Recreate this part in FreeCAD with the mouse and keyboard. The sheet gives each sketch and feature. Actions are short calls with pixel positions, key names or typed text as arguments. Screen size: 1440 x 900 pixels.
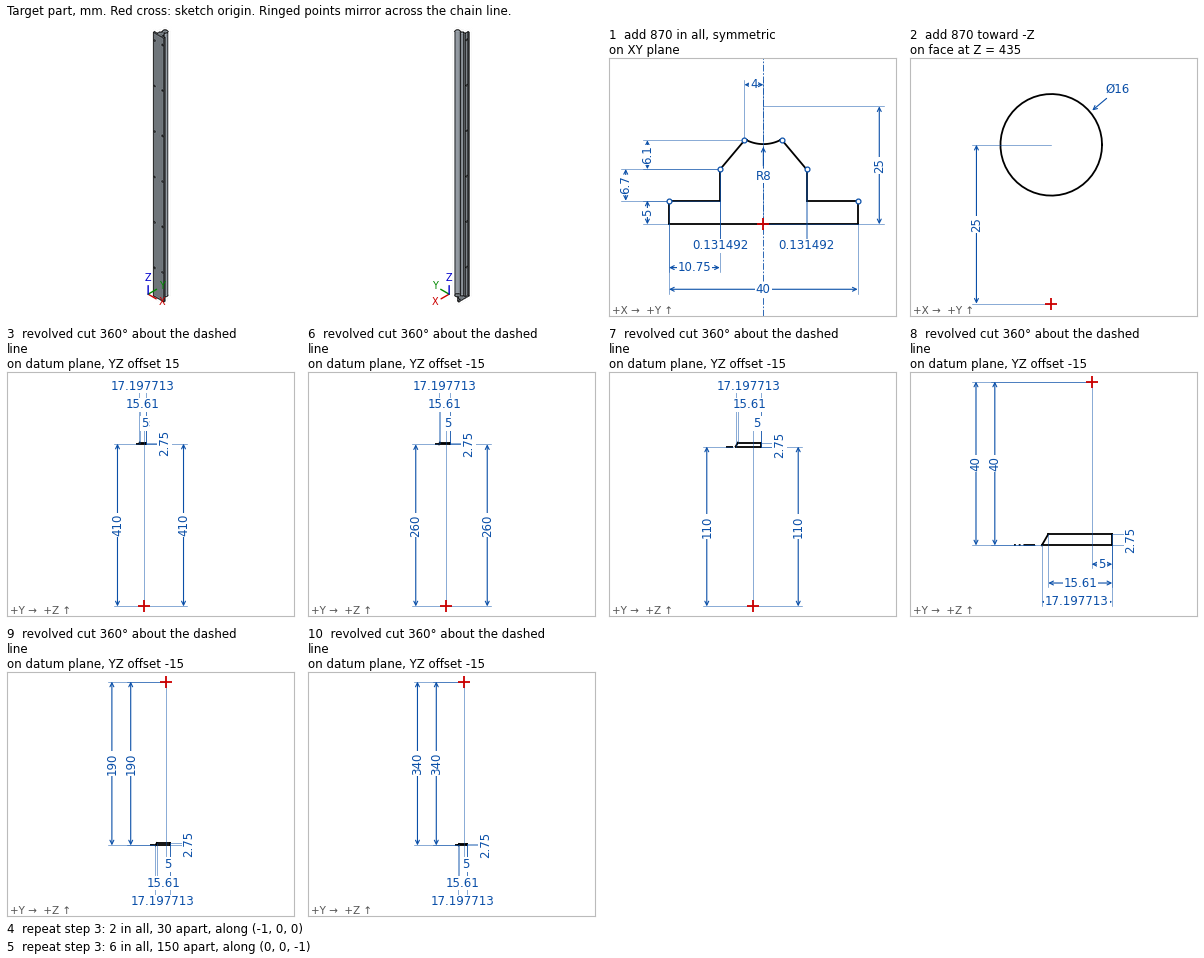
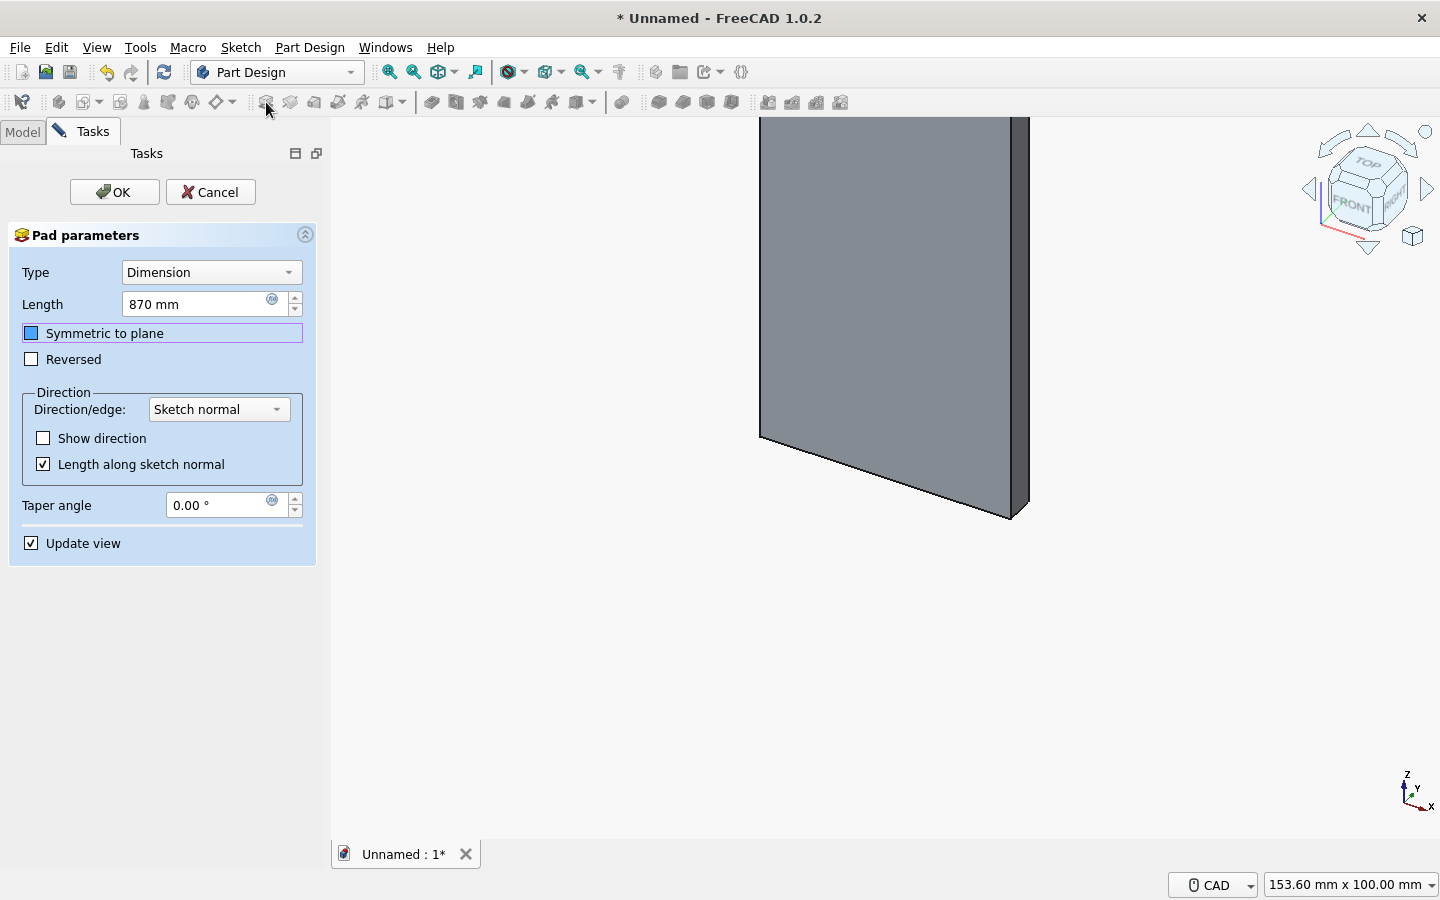
click(30, 333)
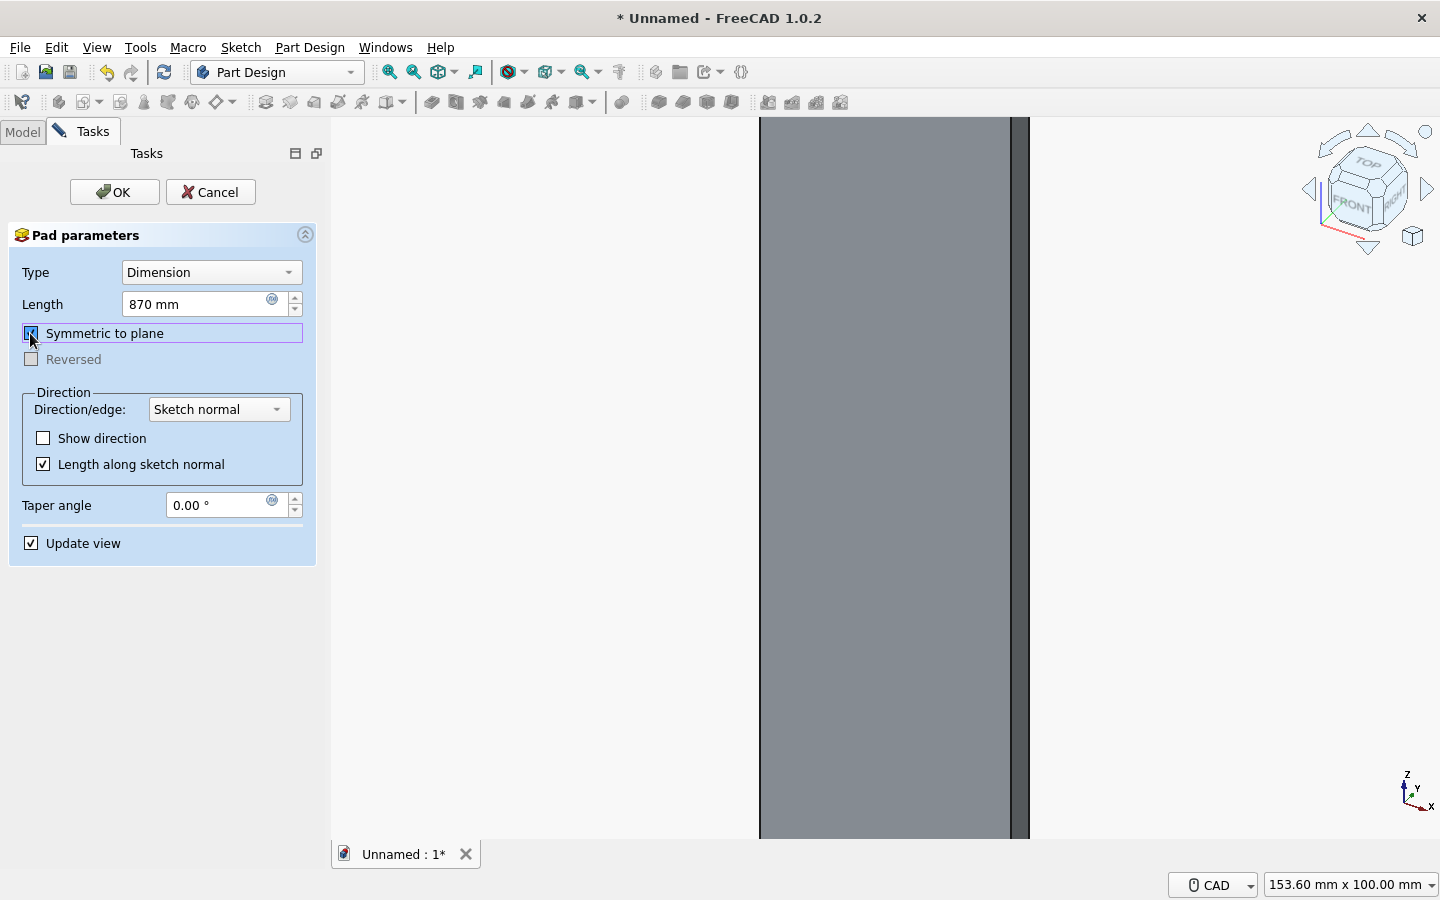
click(115, 192)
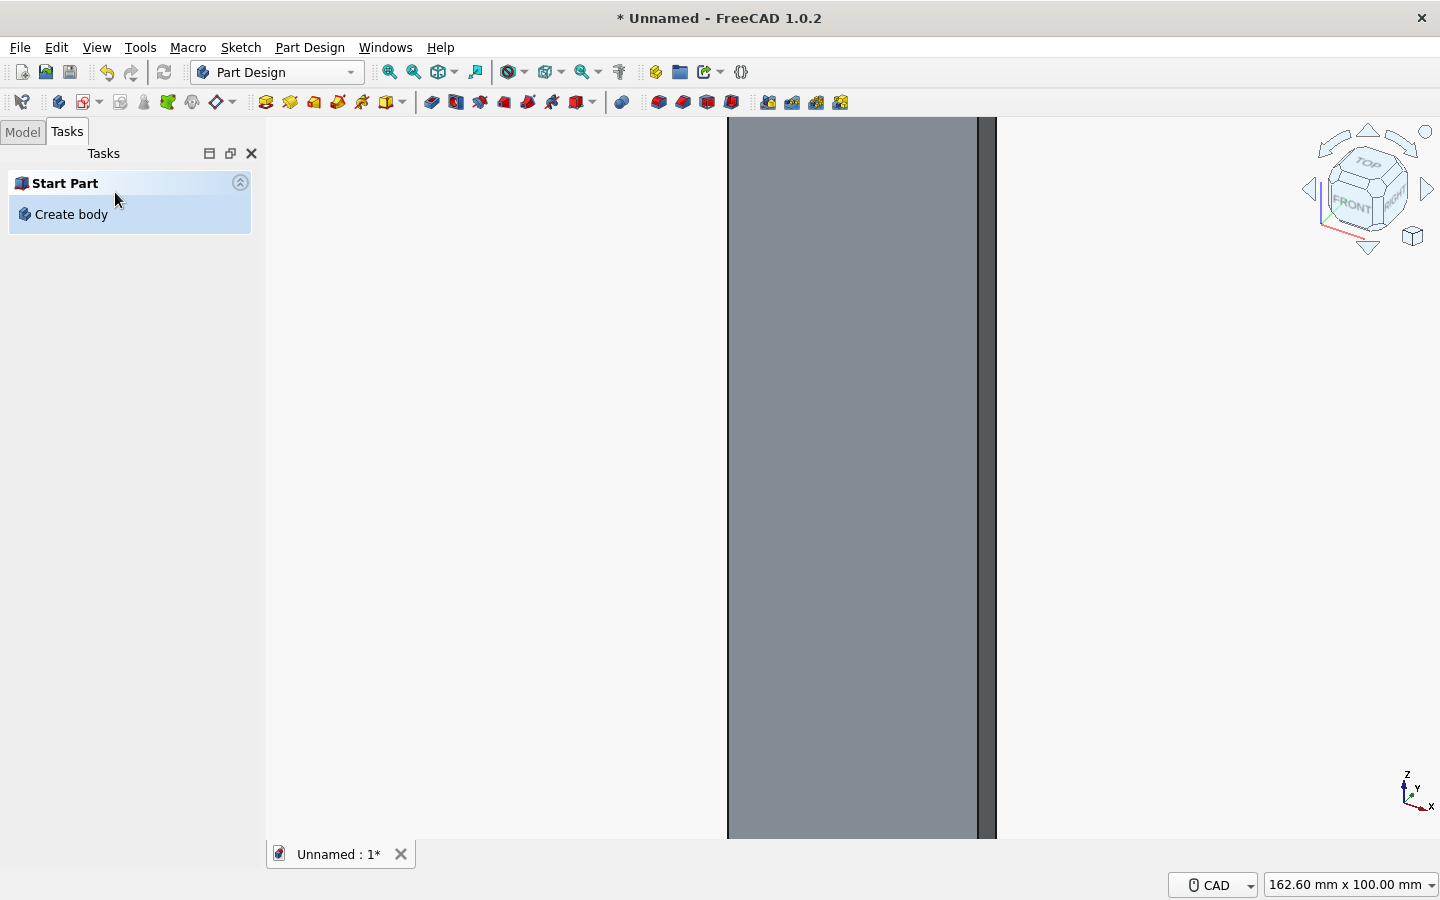
click(390, 72)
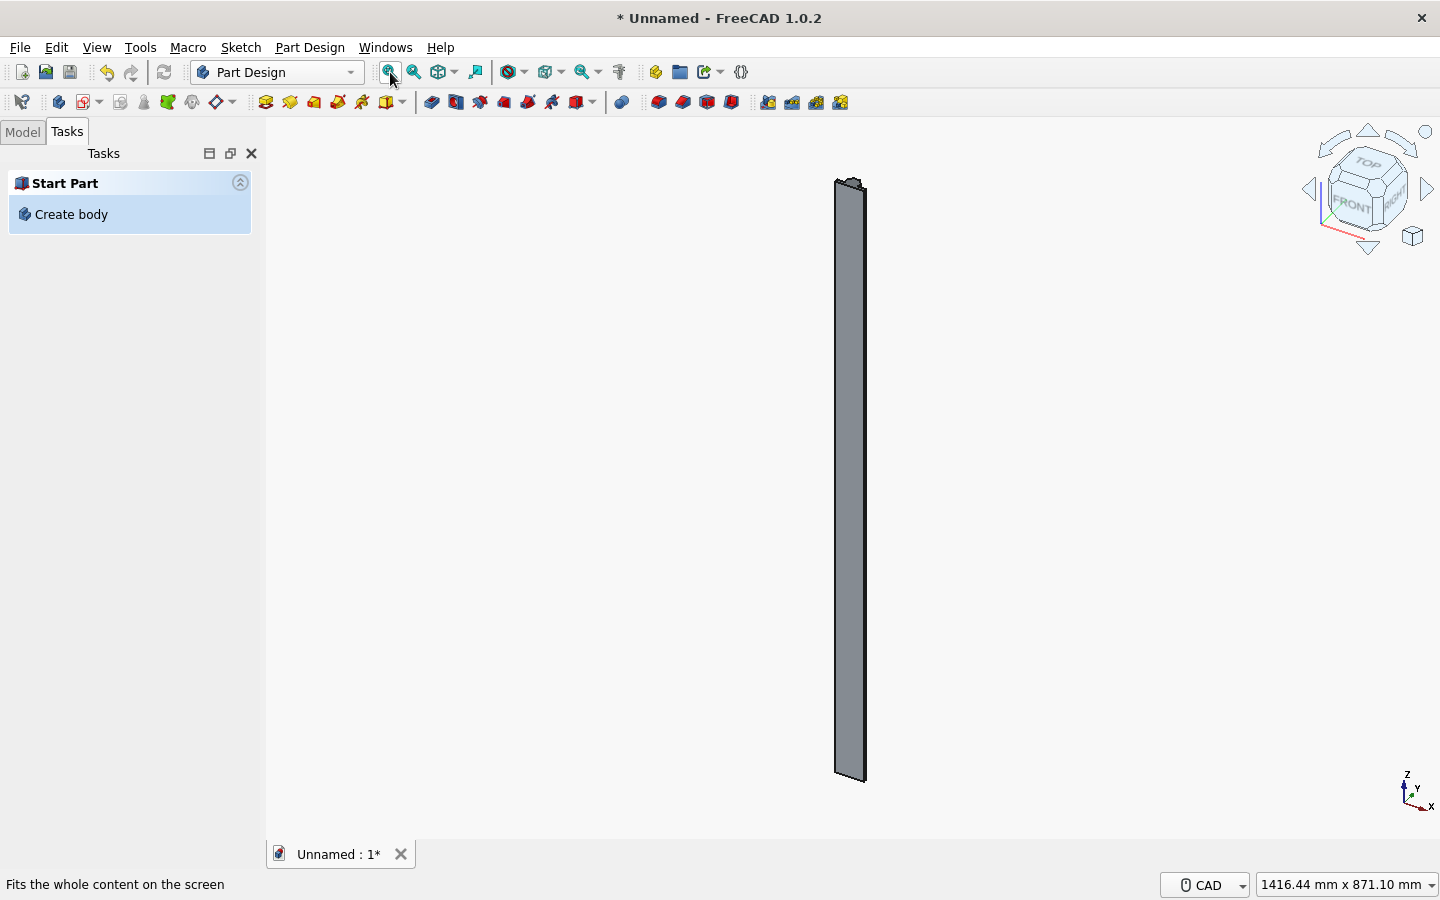
scroll(853, 182, up, 3)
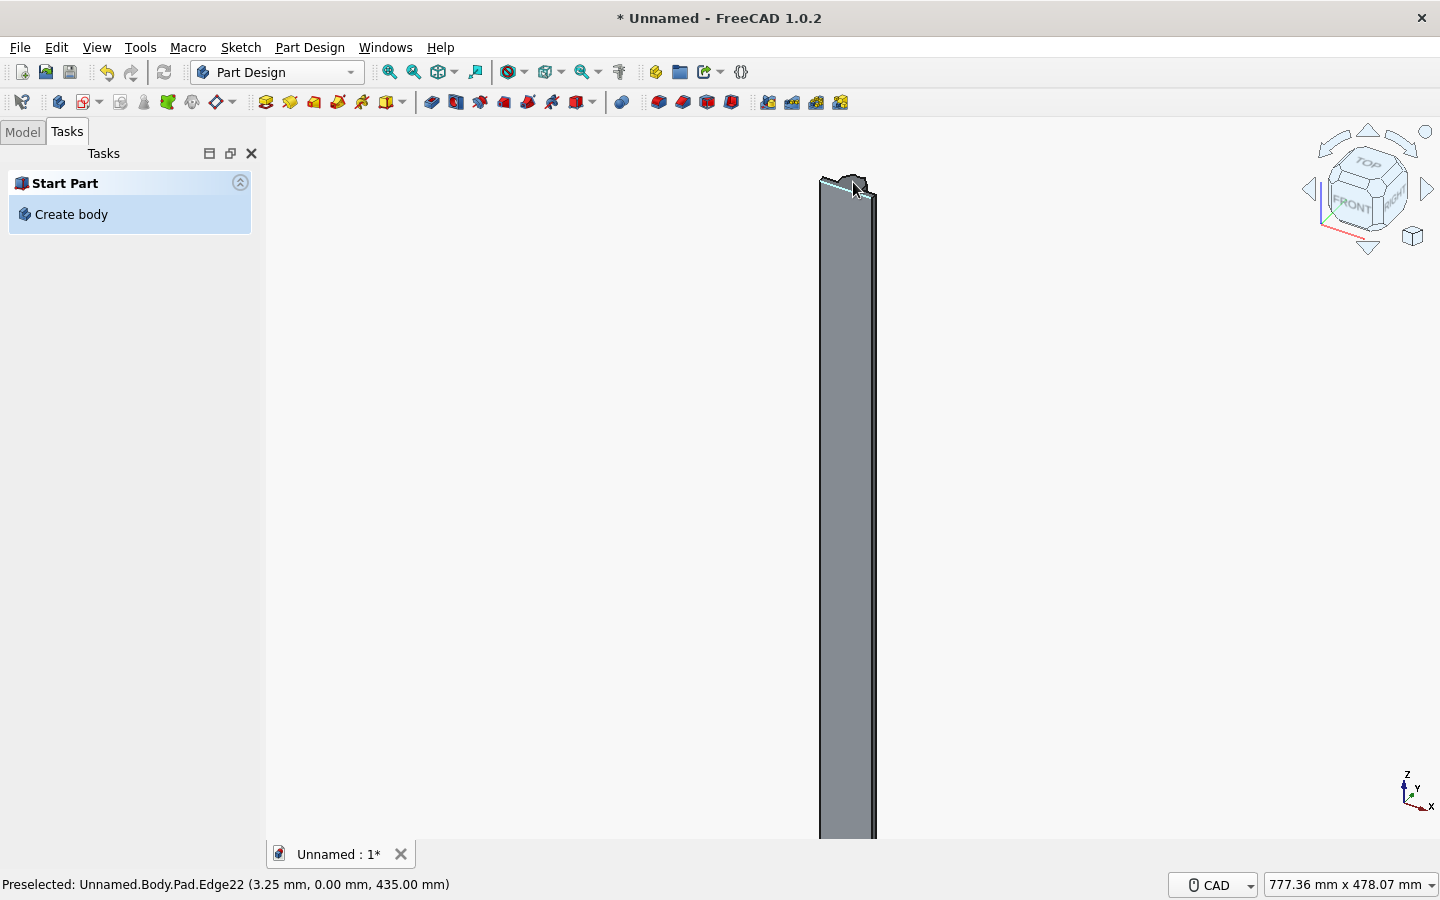
click(855, 180)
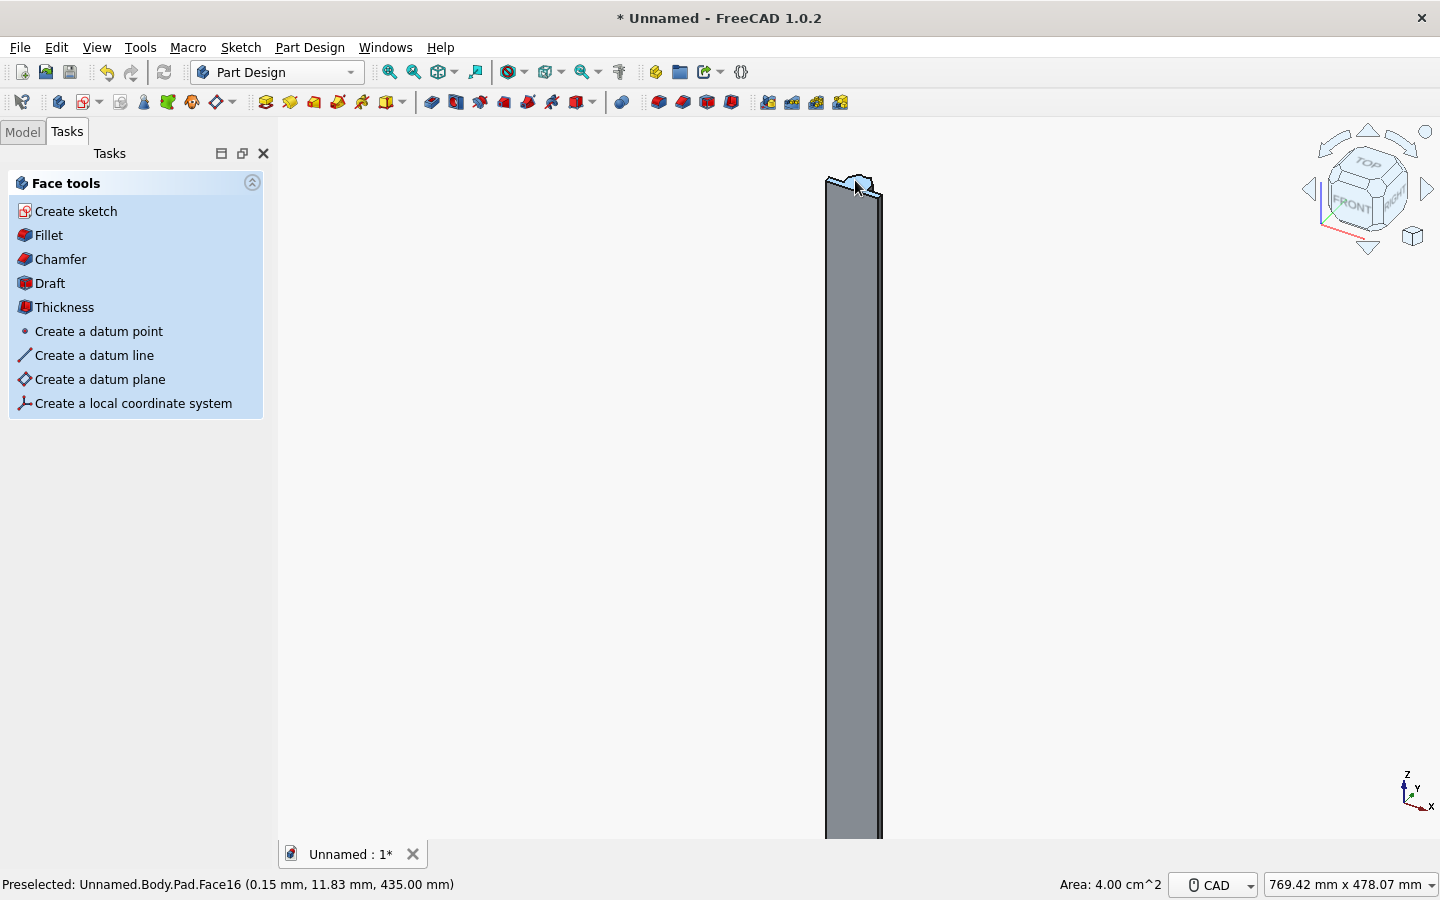
click(84, 102)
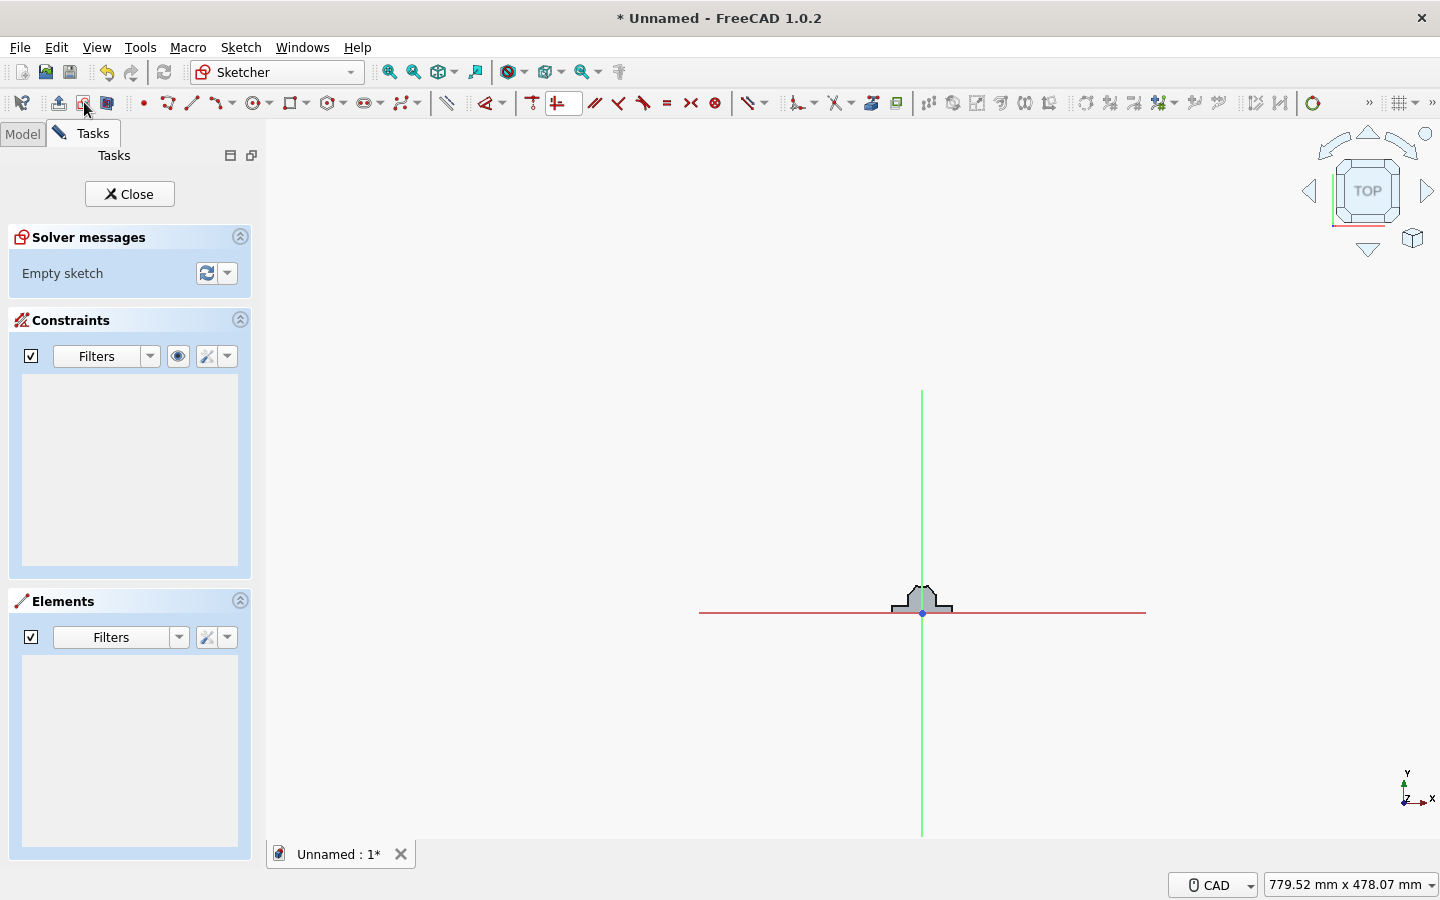
scroll(939, 602, up, 11)